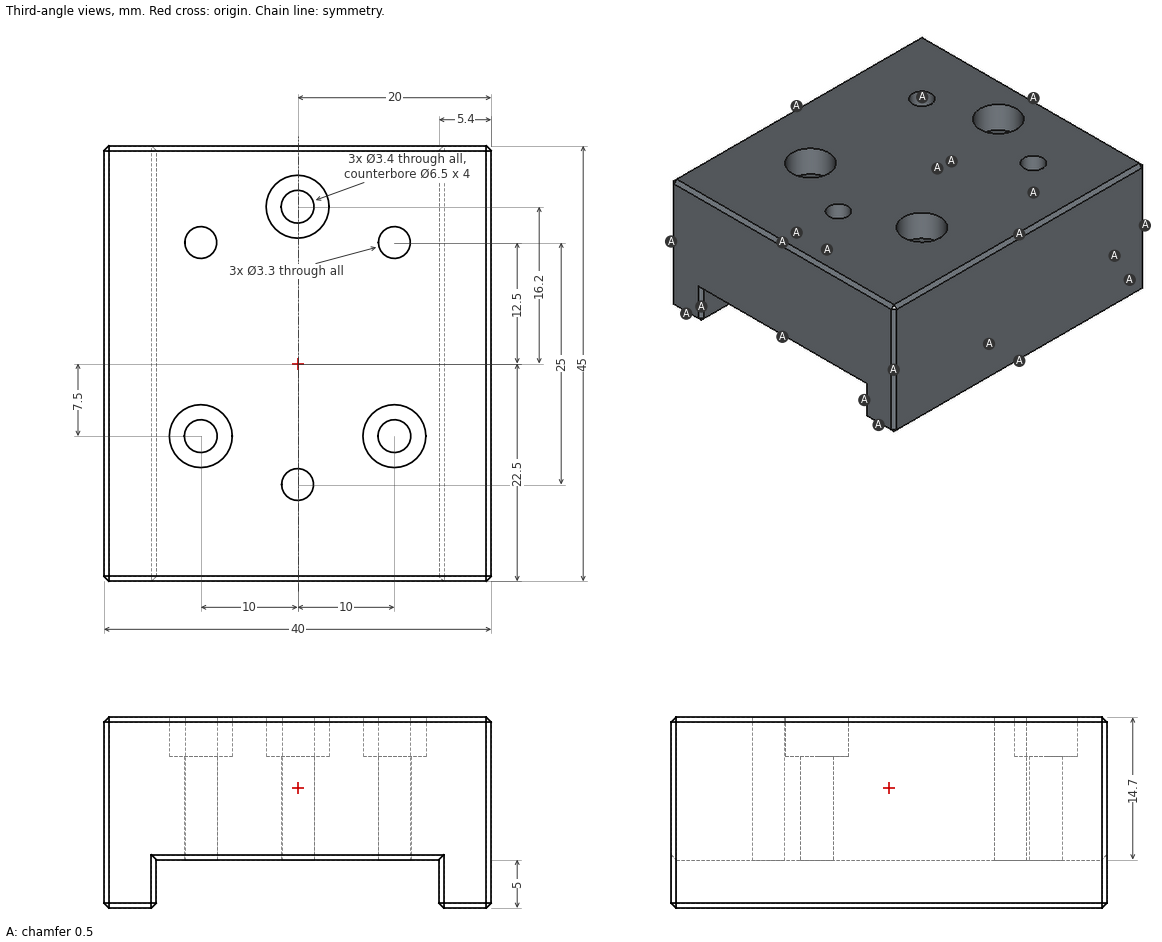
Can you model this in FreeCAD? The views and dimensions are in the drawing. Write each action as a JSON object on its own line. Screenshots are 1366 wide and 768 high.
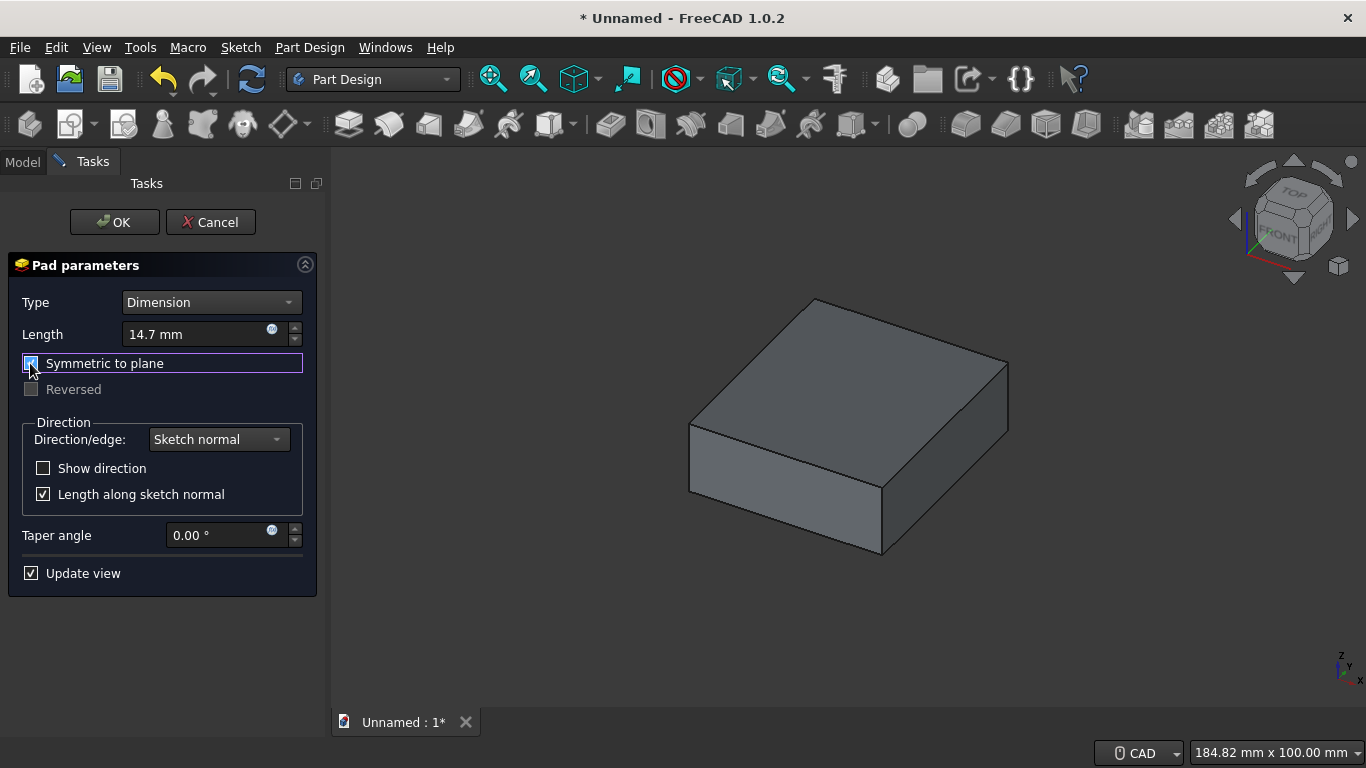
{"action": "left_click", "coordinate": [115, 222]}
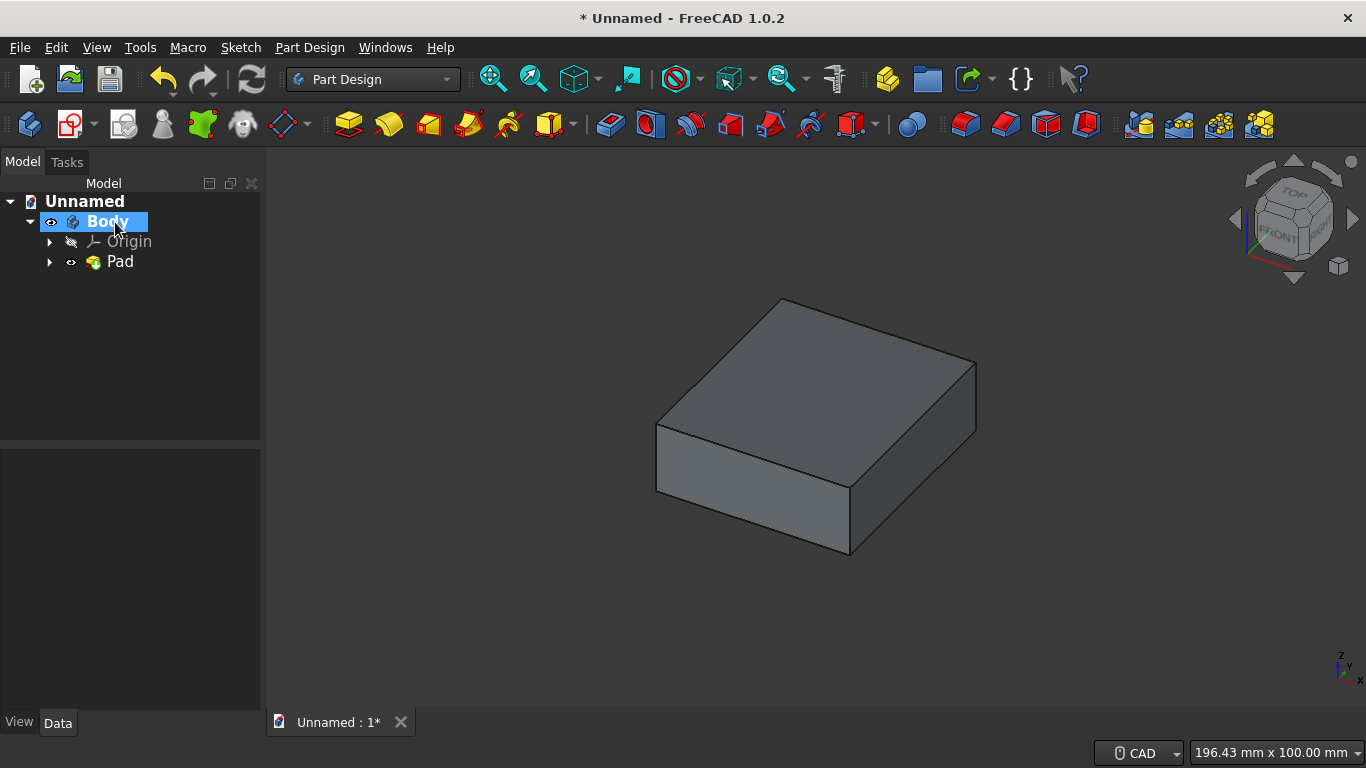
{"action": "left_click", "coordinate": [816, 392]}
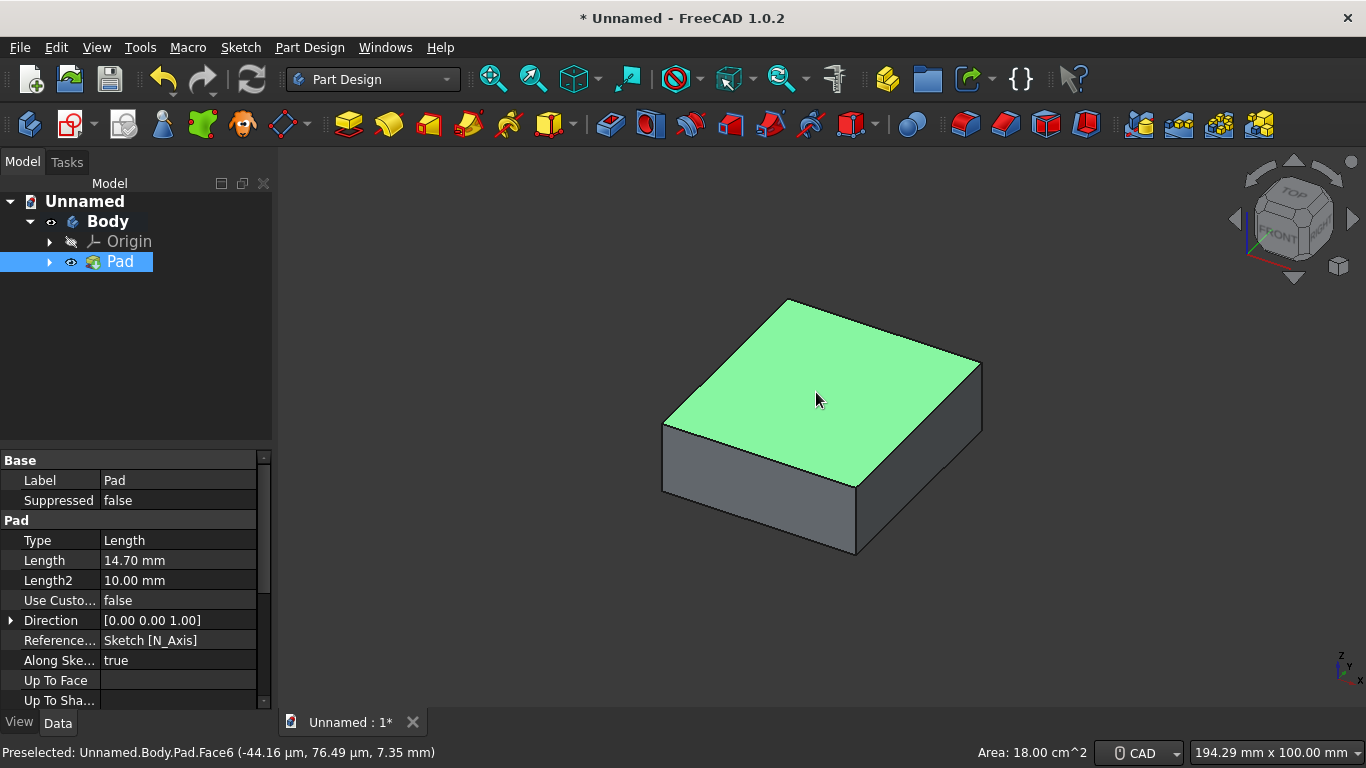
{"action": "left_click", "coordinate": [70, 124]}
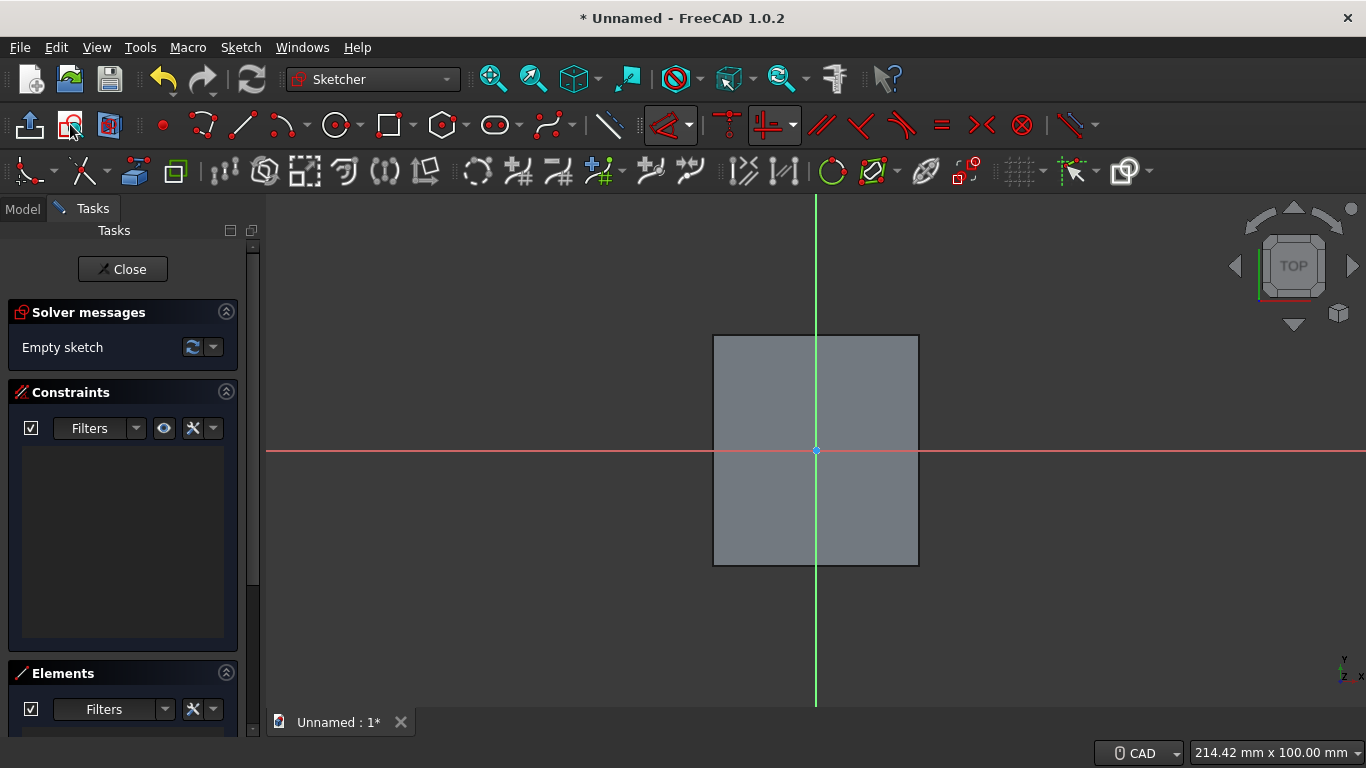
{"action": "scroll", "coordinate": [872, 410], "scroll_direction": "up", "scroll_amount": 4}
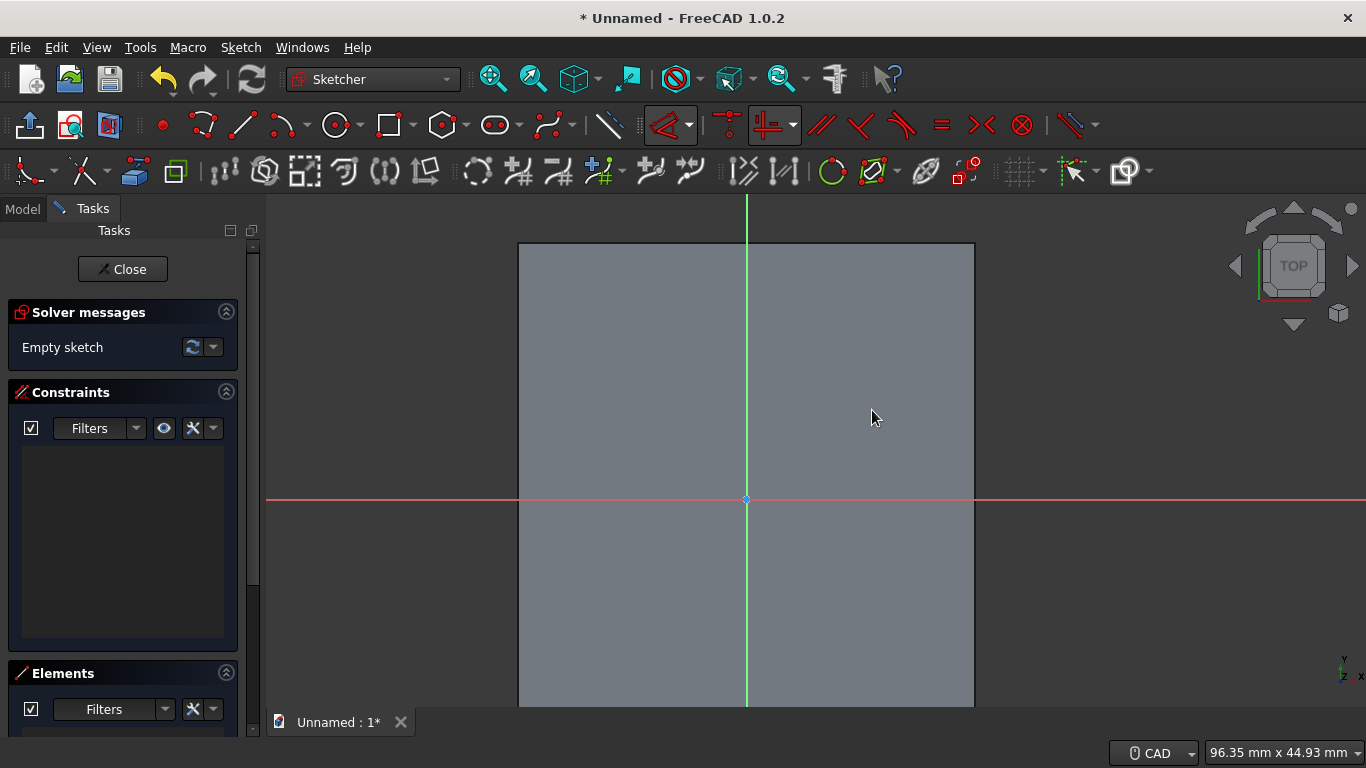
{"action": "left_click", "coordinate": [336, 126]}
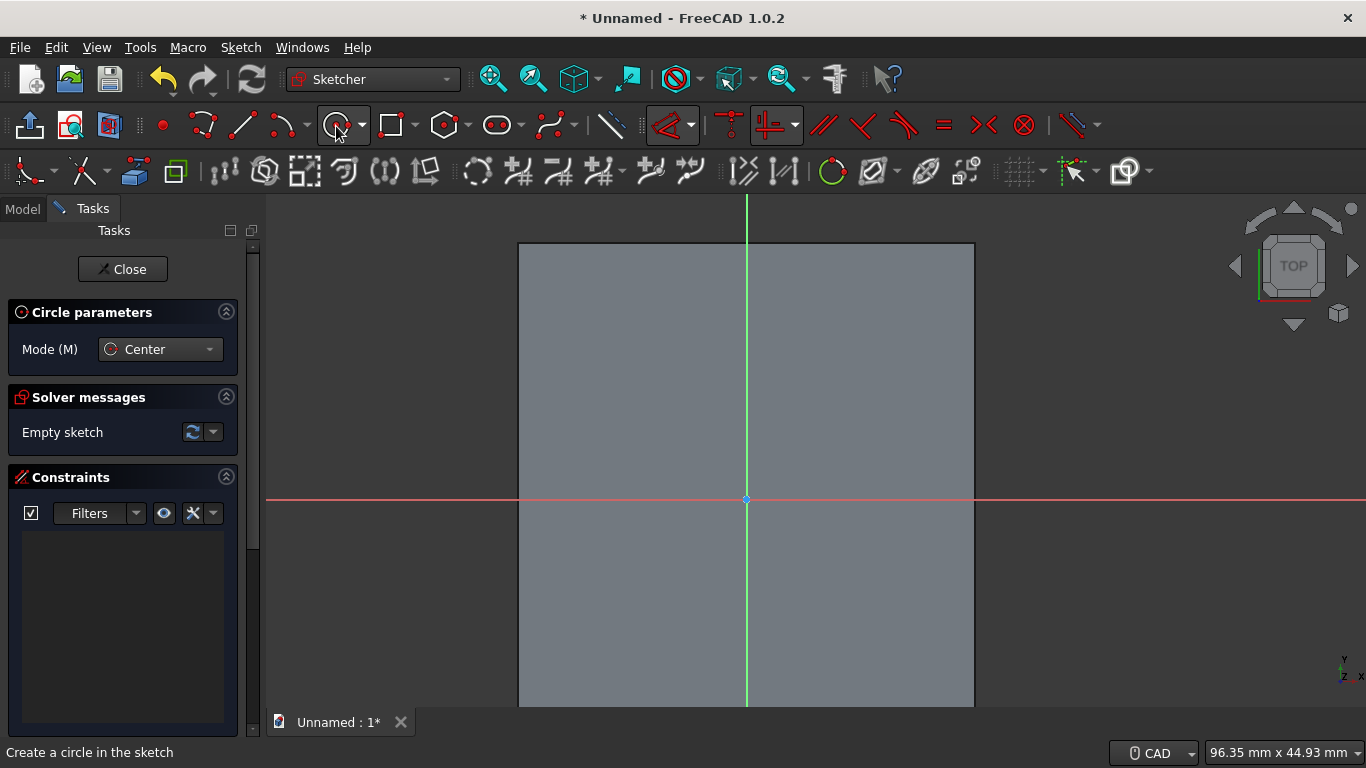
{"action": "left_click", "coordinate": [747, 315]}
{"action": "left_click", "coordinate": [765, 308]}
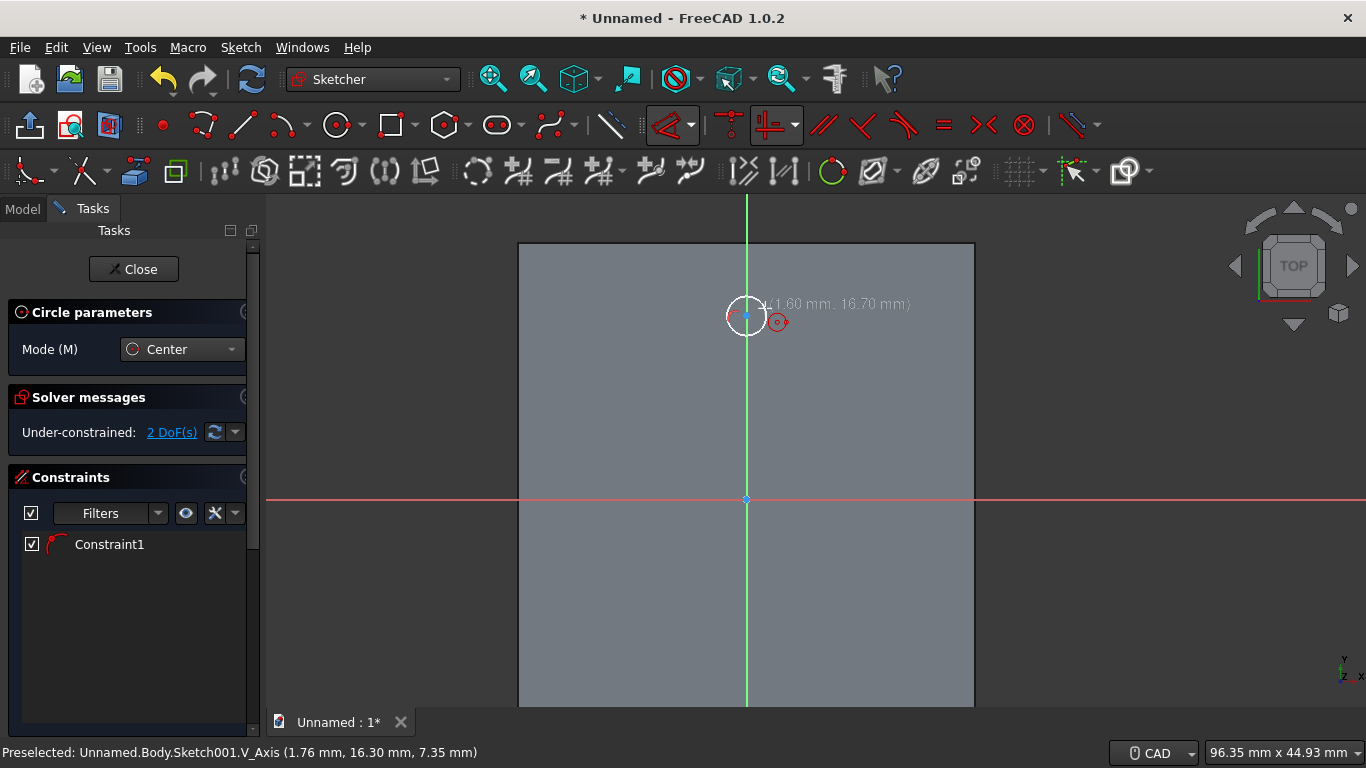
{"action": "left_click", "coordinate": [633, 585]}
{"action": "left_click", "coordinate": [646, 572]}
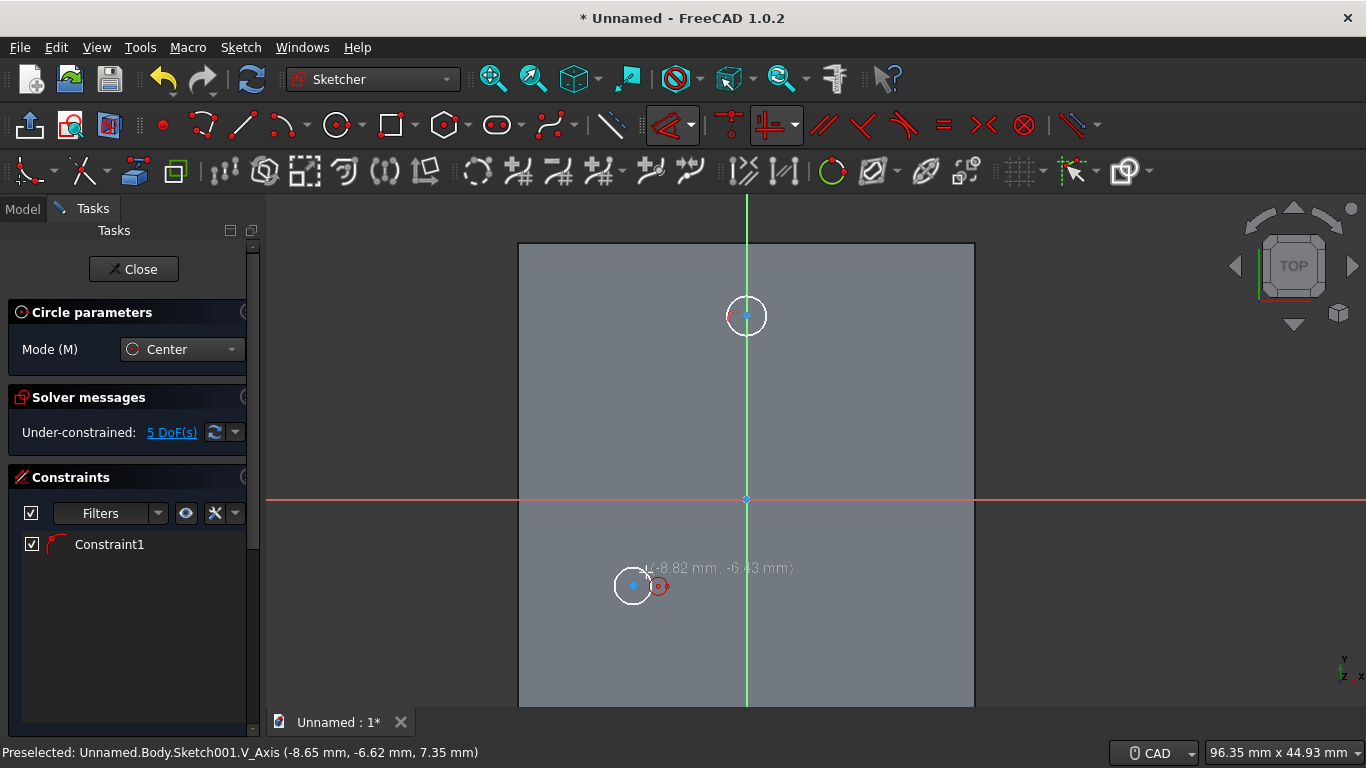
{"action": "left_click", "coordinate": [861, 585]}
{"action": "left_click", "coordinate": [875, 572]}
{"action": "key", "text": "Escape"}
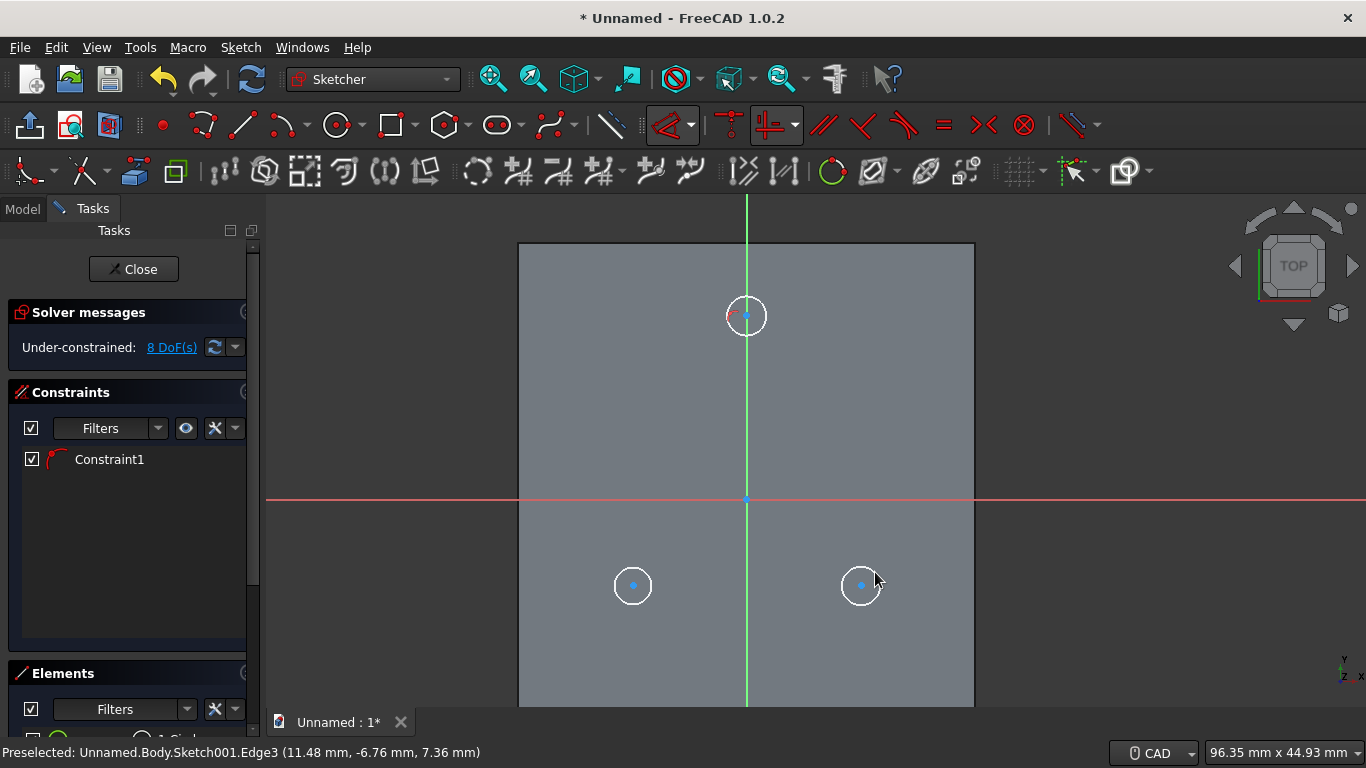
{"action": "left_click", "coordinate": [761, 302]}